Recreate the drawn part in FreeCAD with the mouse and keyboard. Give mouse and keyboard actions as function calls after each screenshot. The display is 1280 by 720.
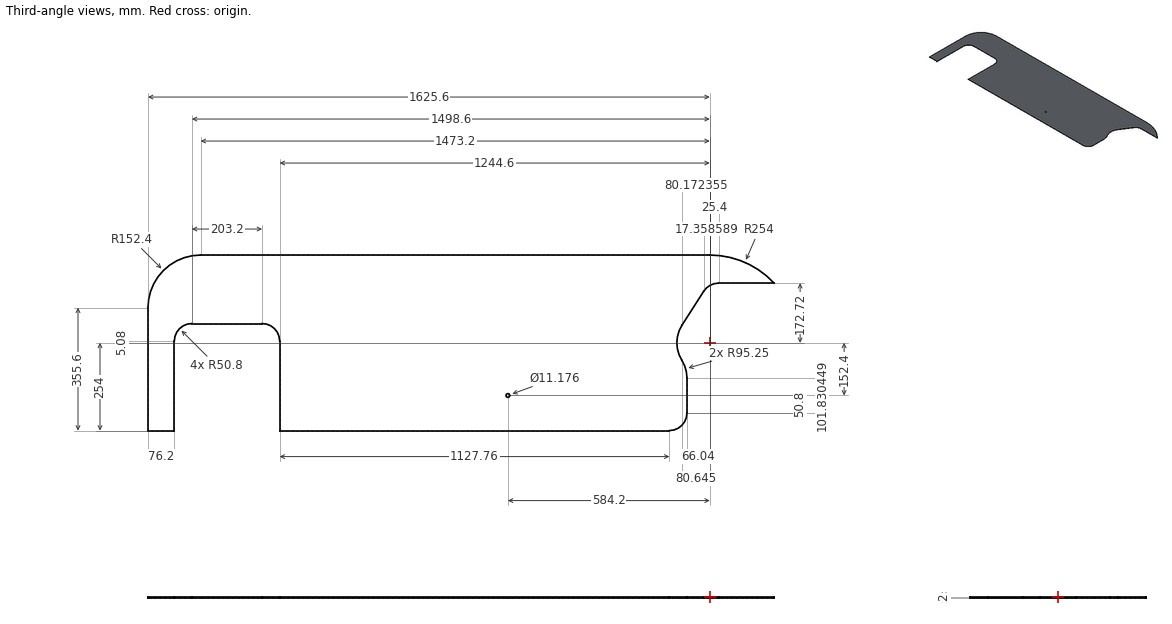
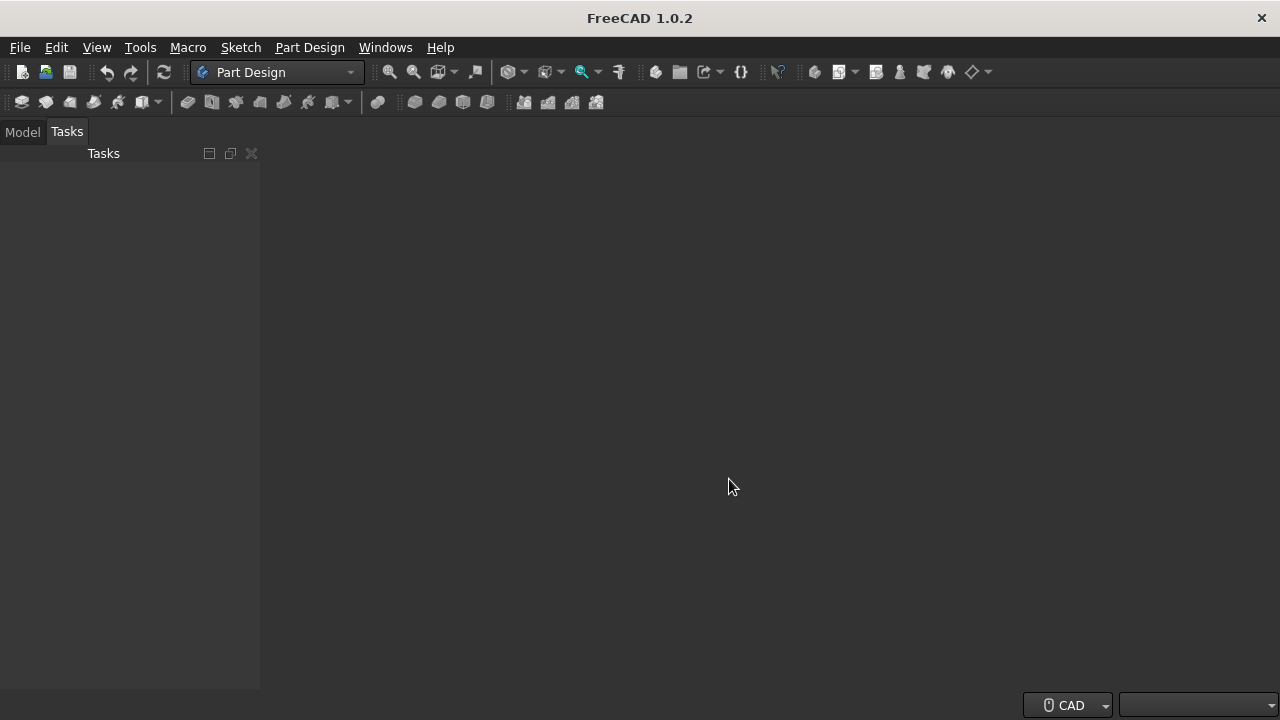
click(22, 72)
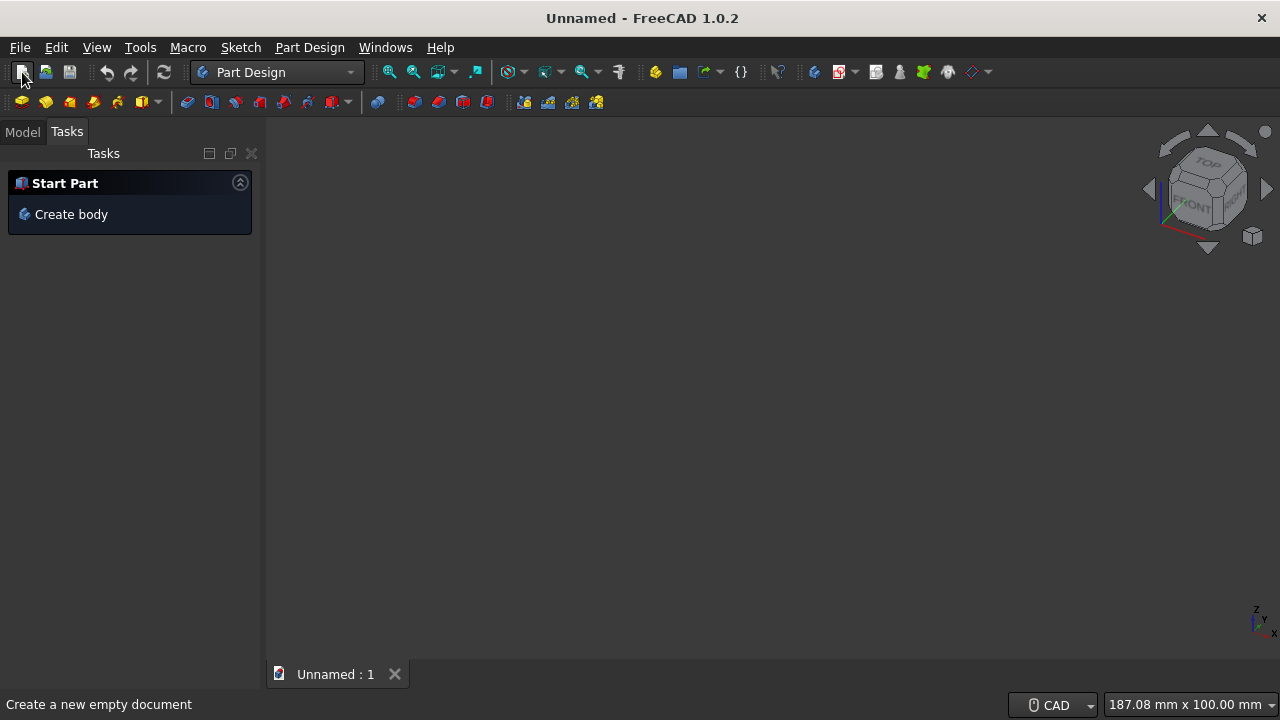
click(840, 72)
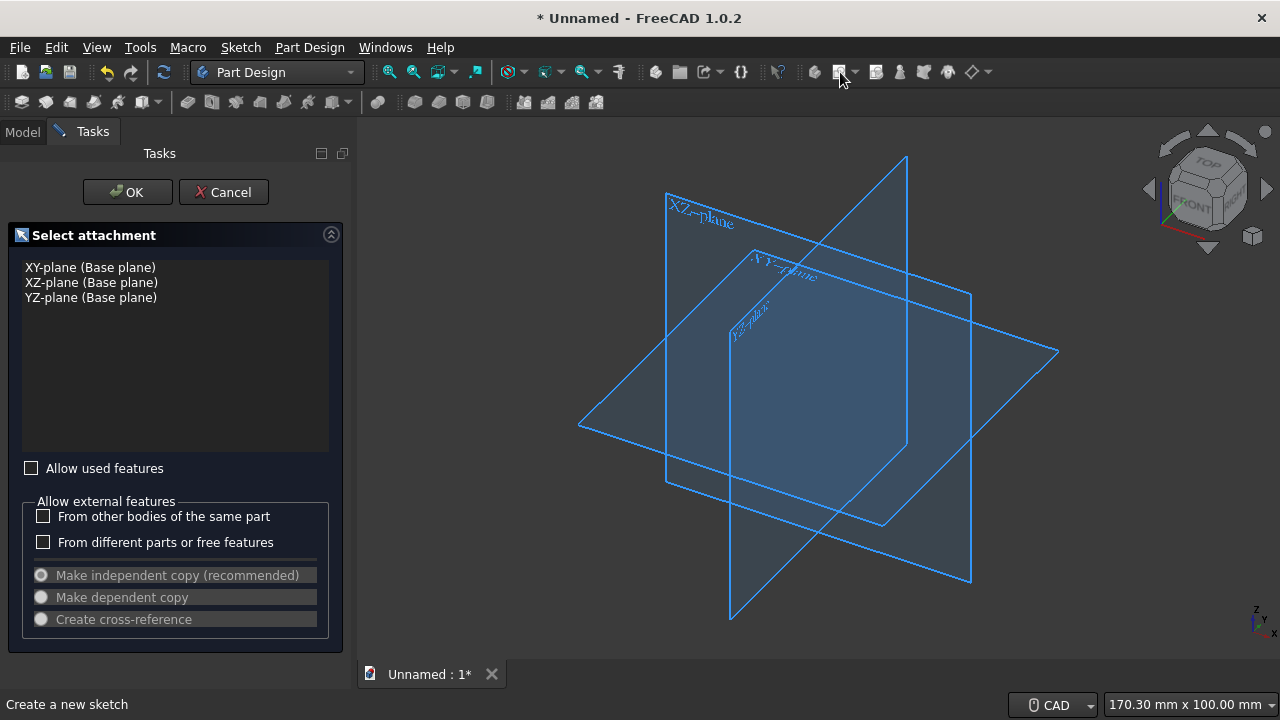
click(82, 268)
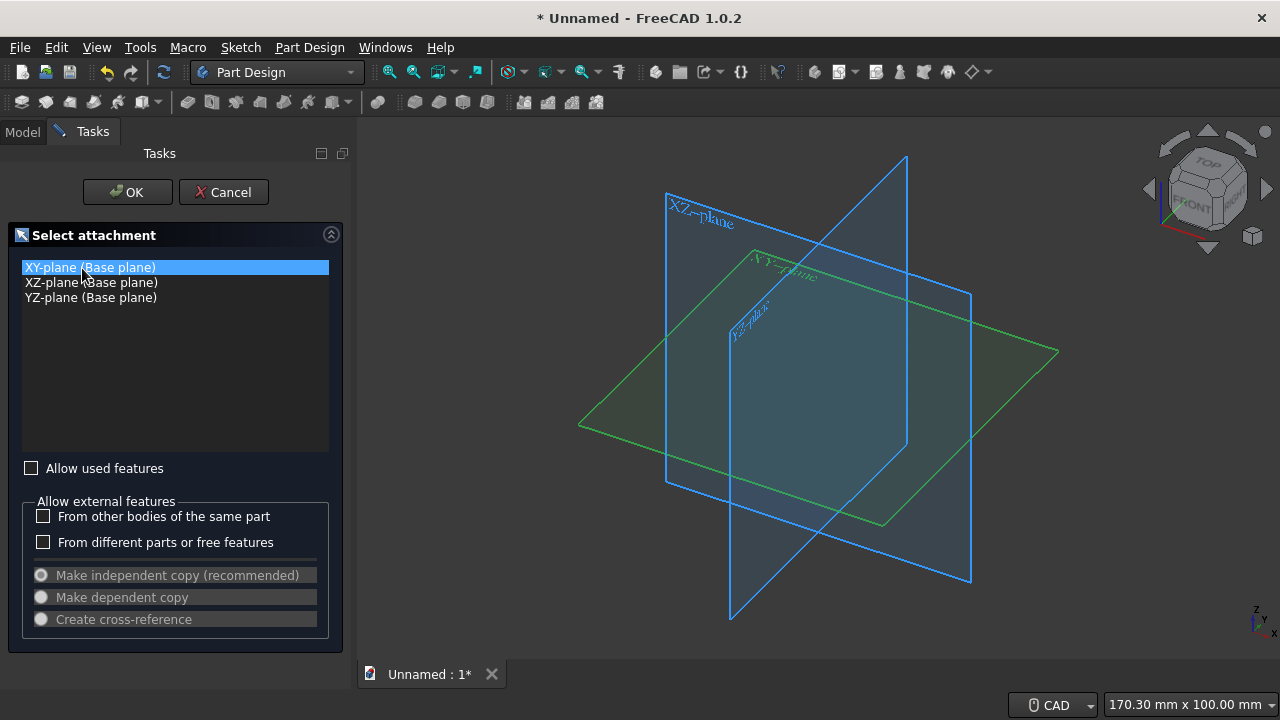
click(128, 192)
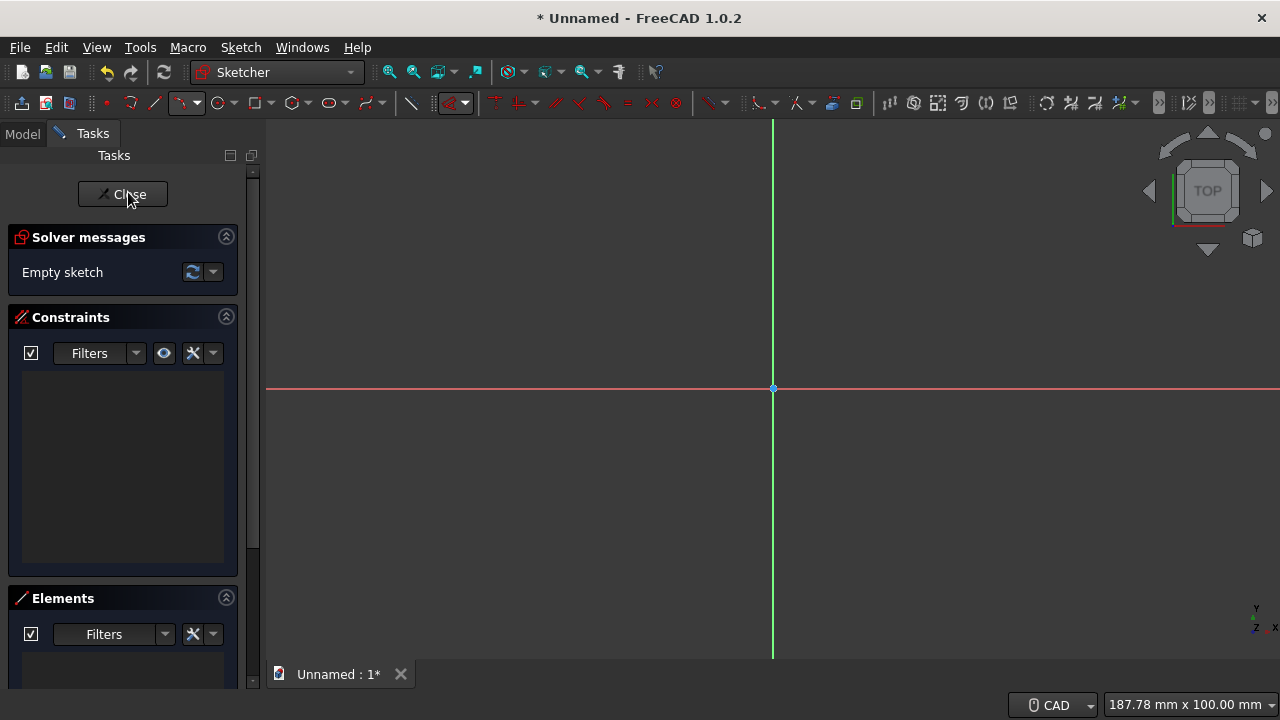
scroll(952, 389, down, 14)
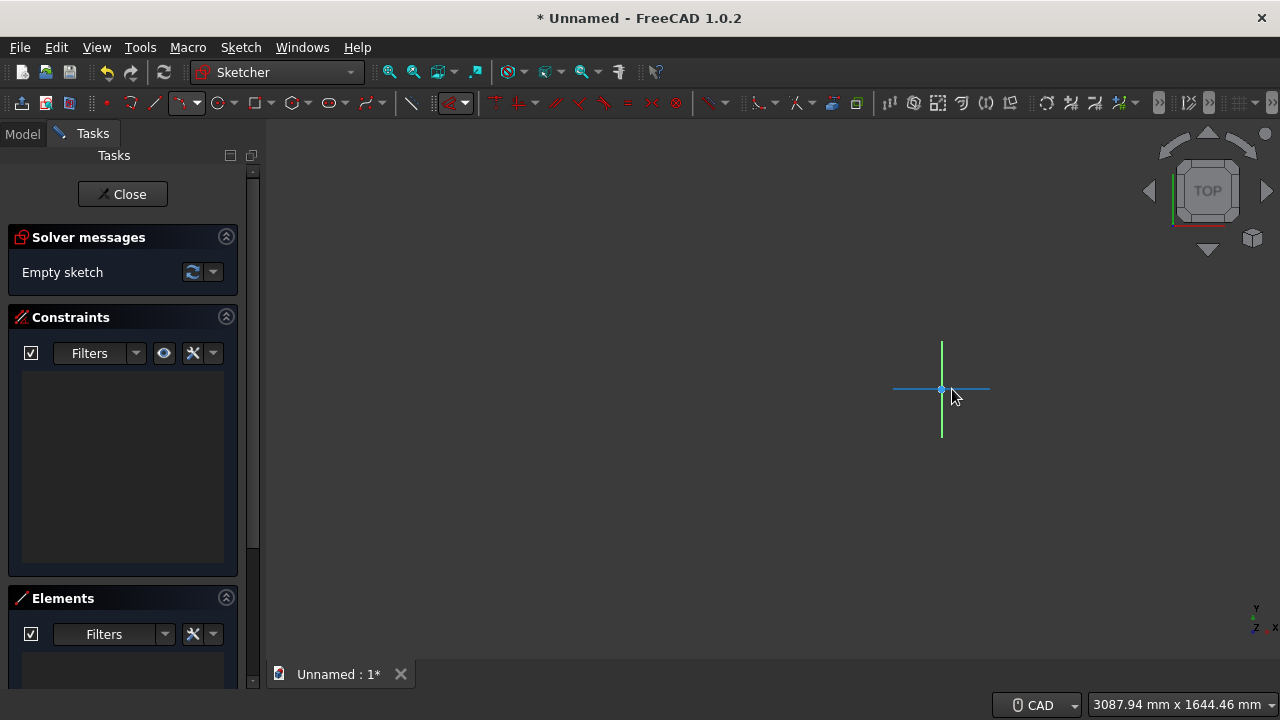
click(156, 104)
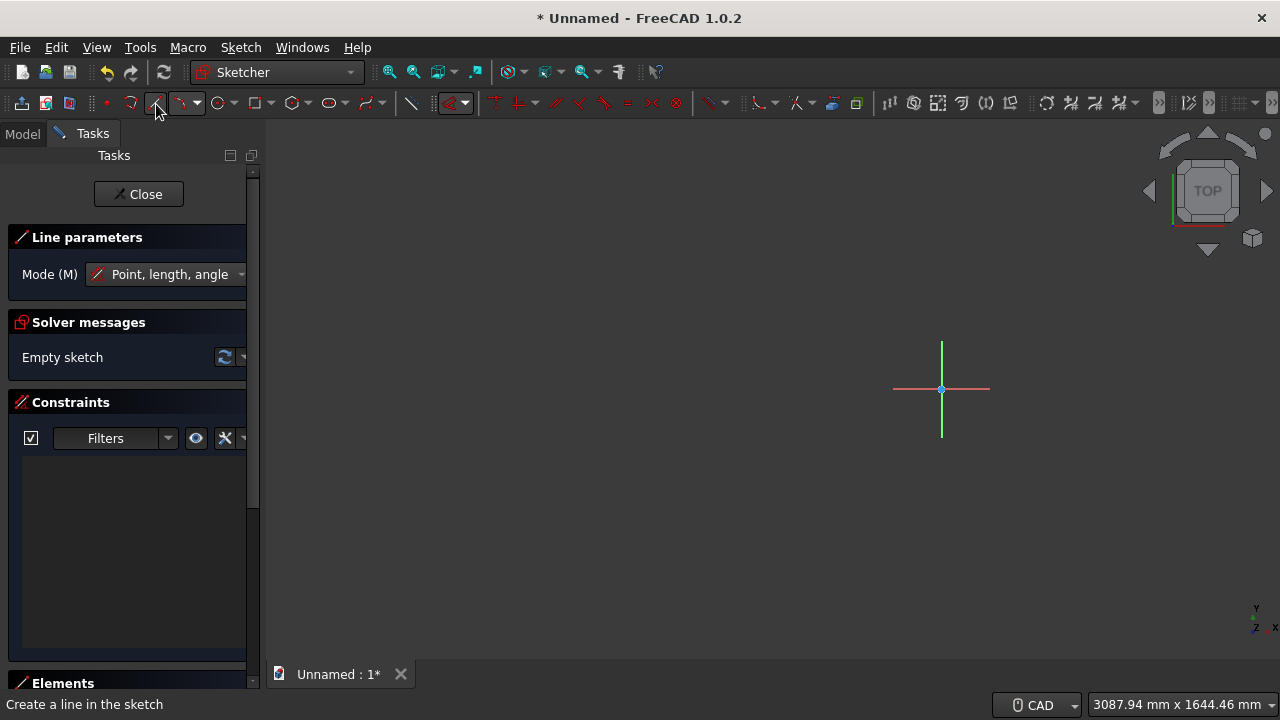
scroll(950, 333, up, 4)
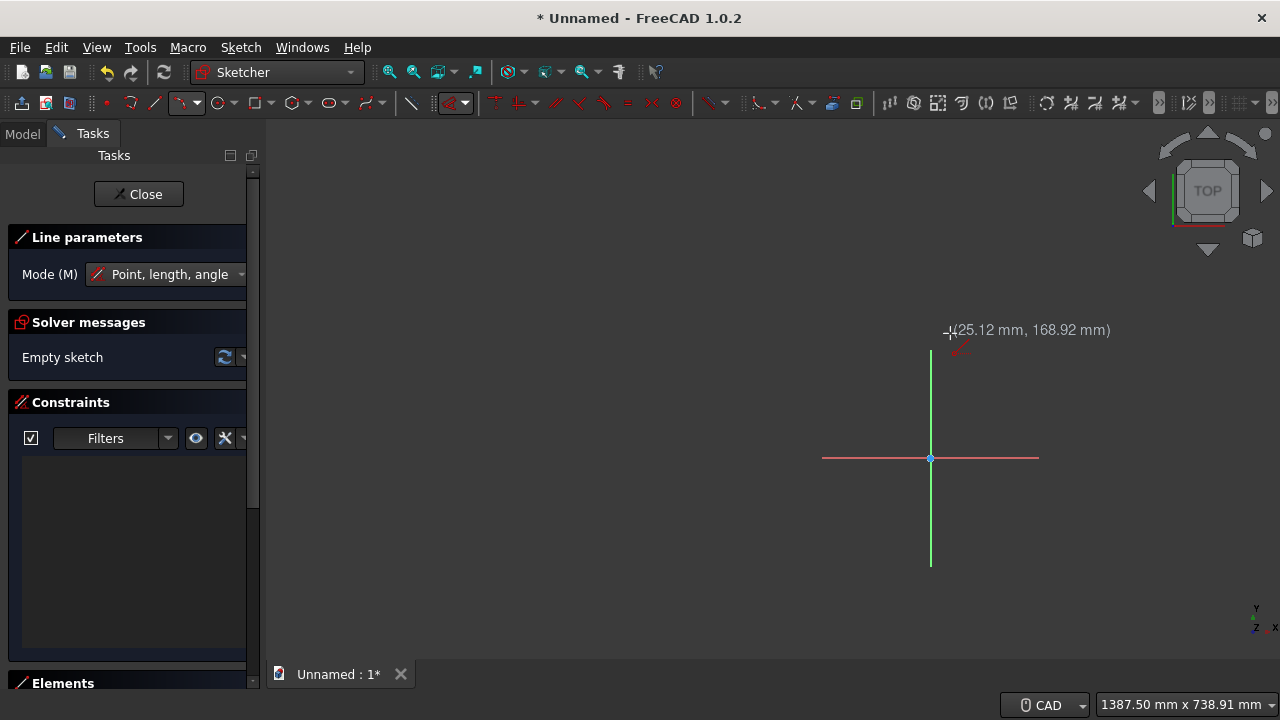
click(949, 332)
click(1067, 332)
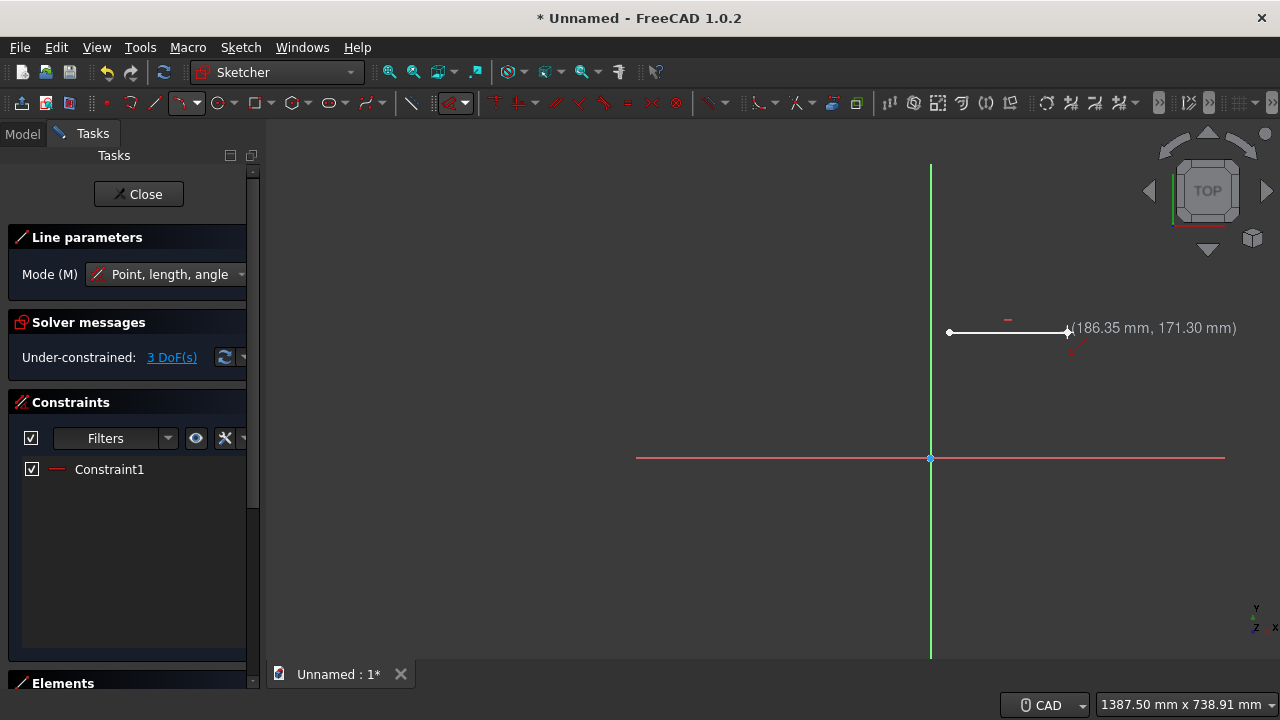
click(931, 273)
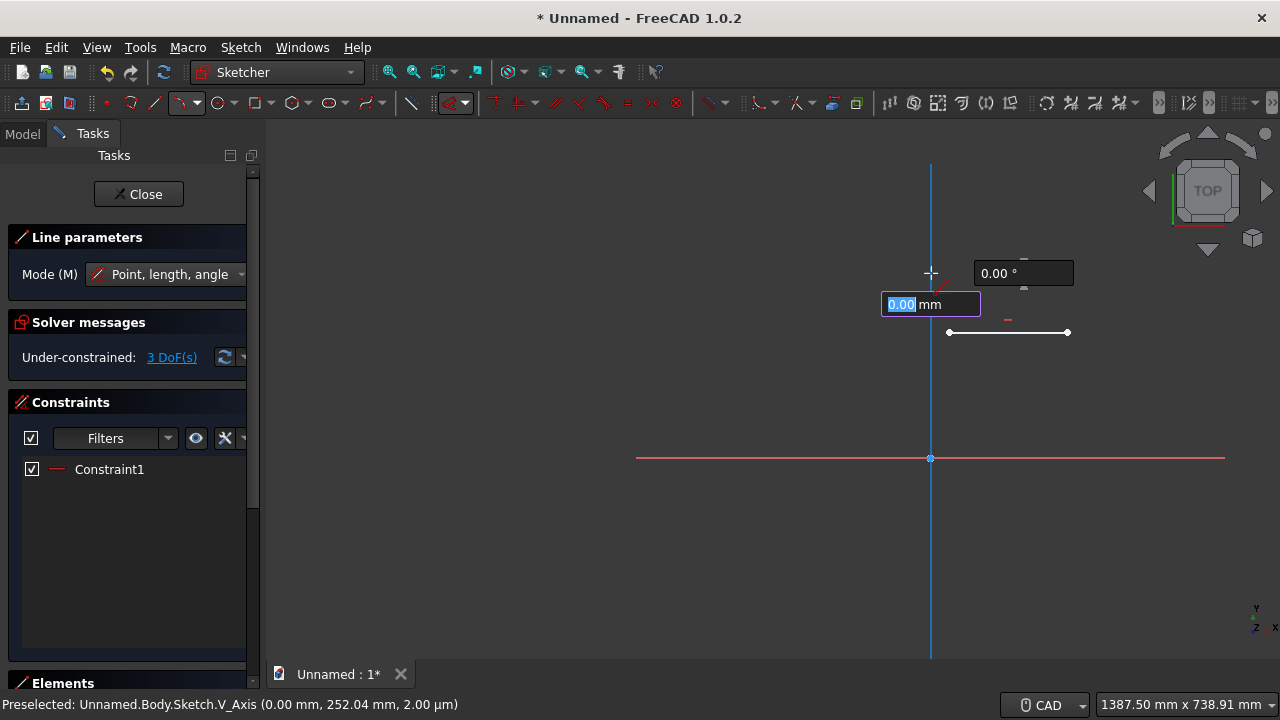
scroll(949, 333, down, 4)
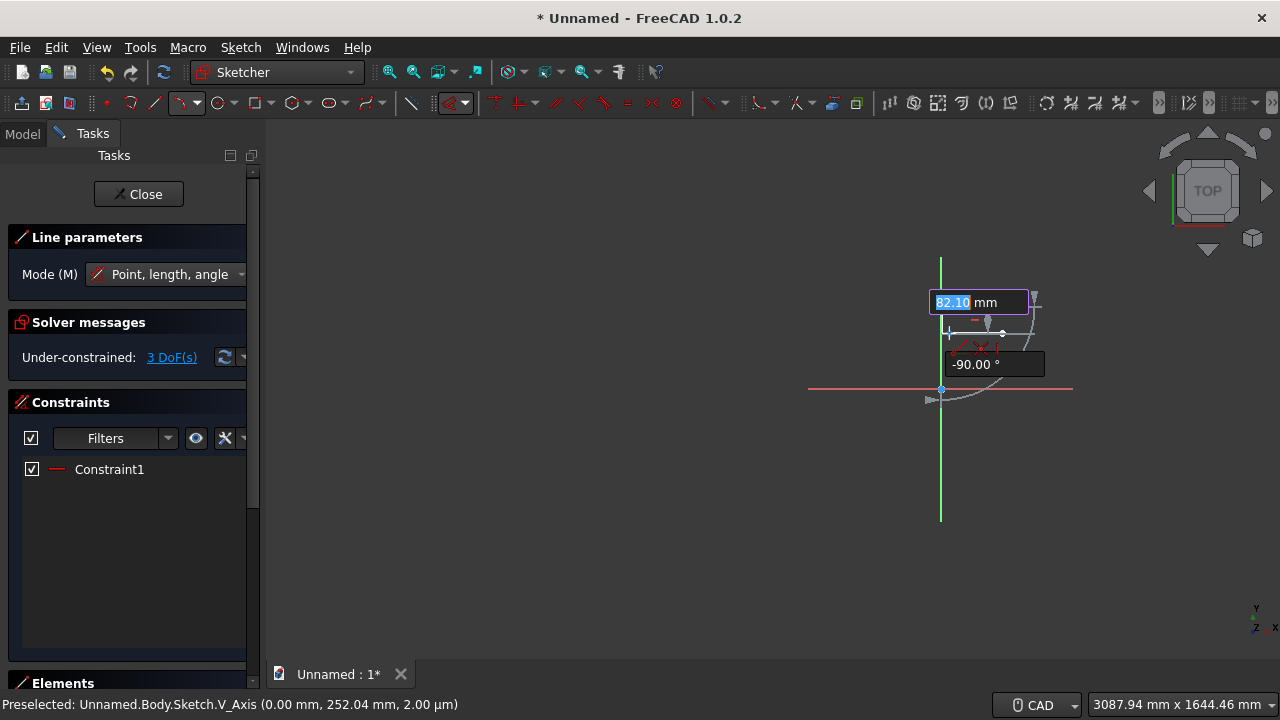
click(457, 306)